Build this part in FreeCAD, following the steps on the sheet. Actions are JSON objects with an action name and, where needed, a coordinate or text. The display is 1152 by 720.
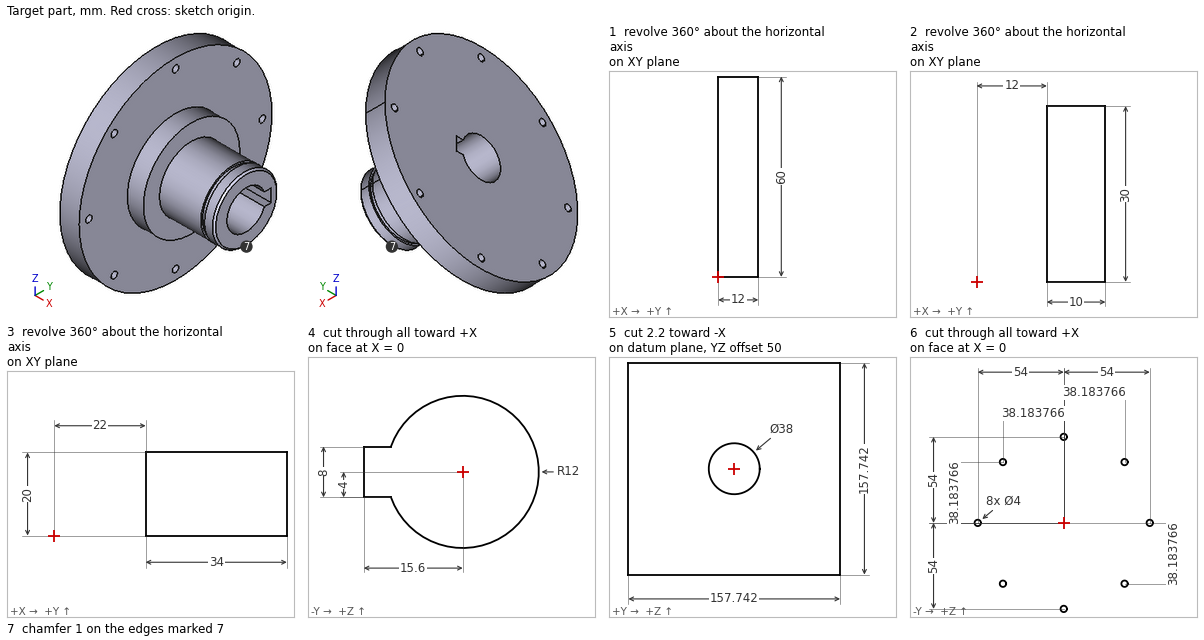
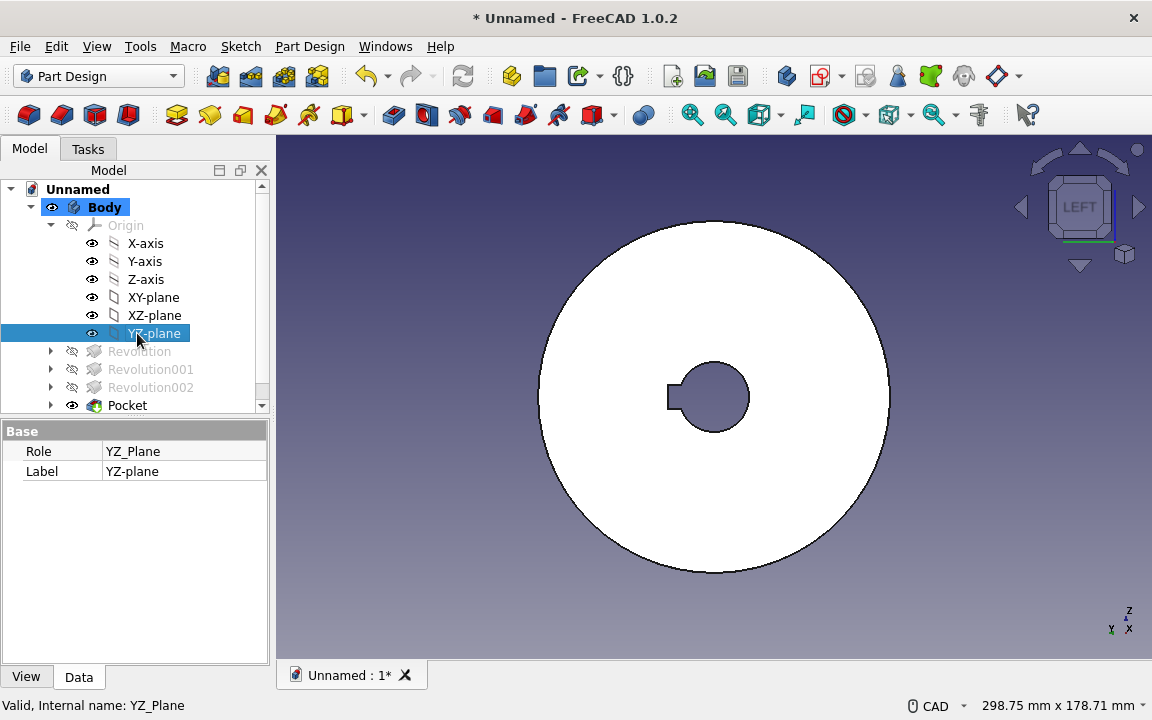
{"action": "left_click", "coordinate": [996, 76]}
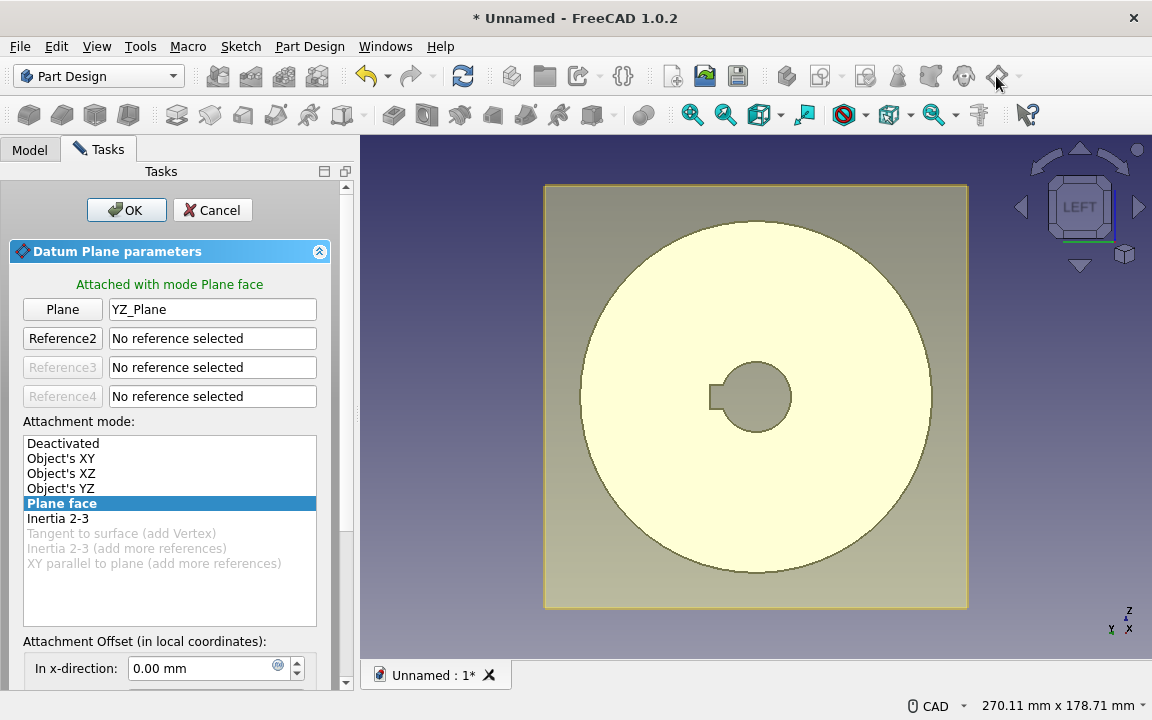
{"action": "scroll", "coordinate": [346, 436], "scroll_direction": "down", "scroll_amount": 2}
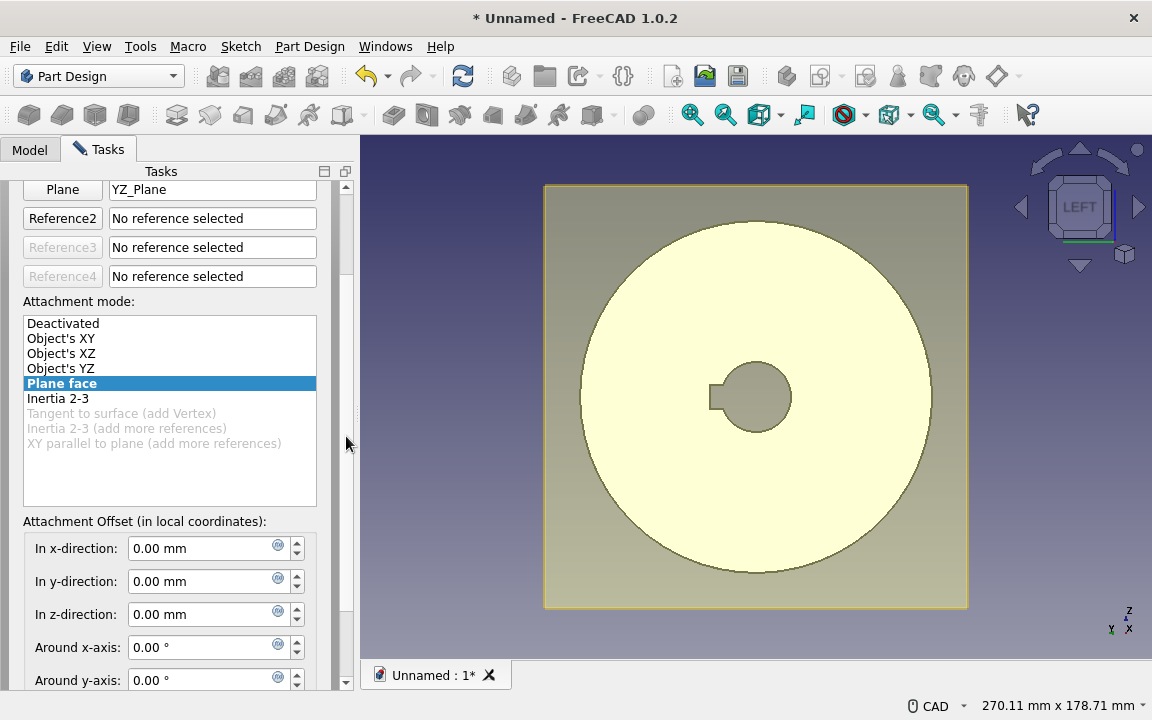
{"action": "triple_click", "coordinate": [210, 614]}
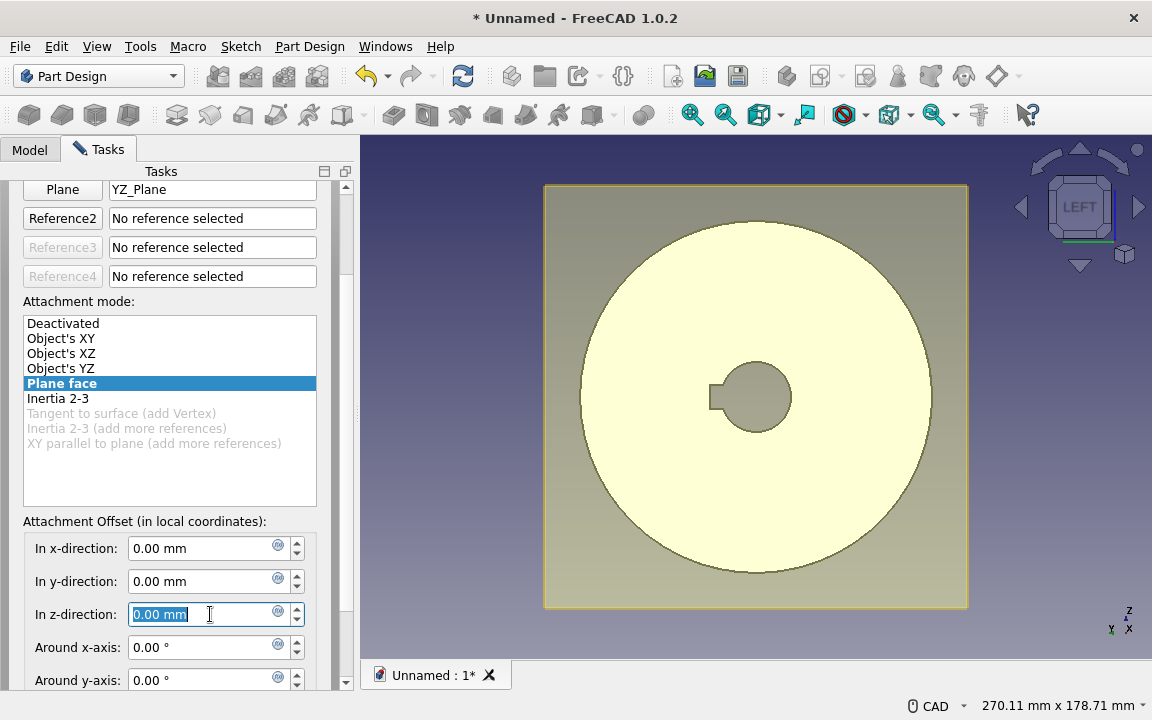
{"action": "type", "text": "50"}
{"action": "key", "text": "Tab"}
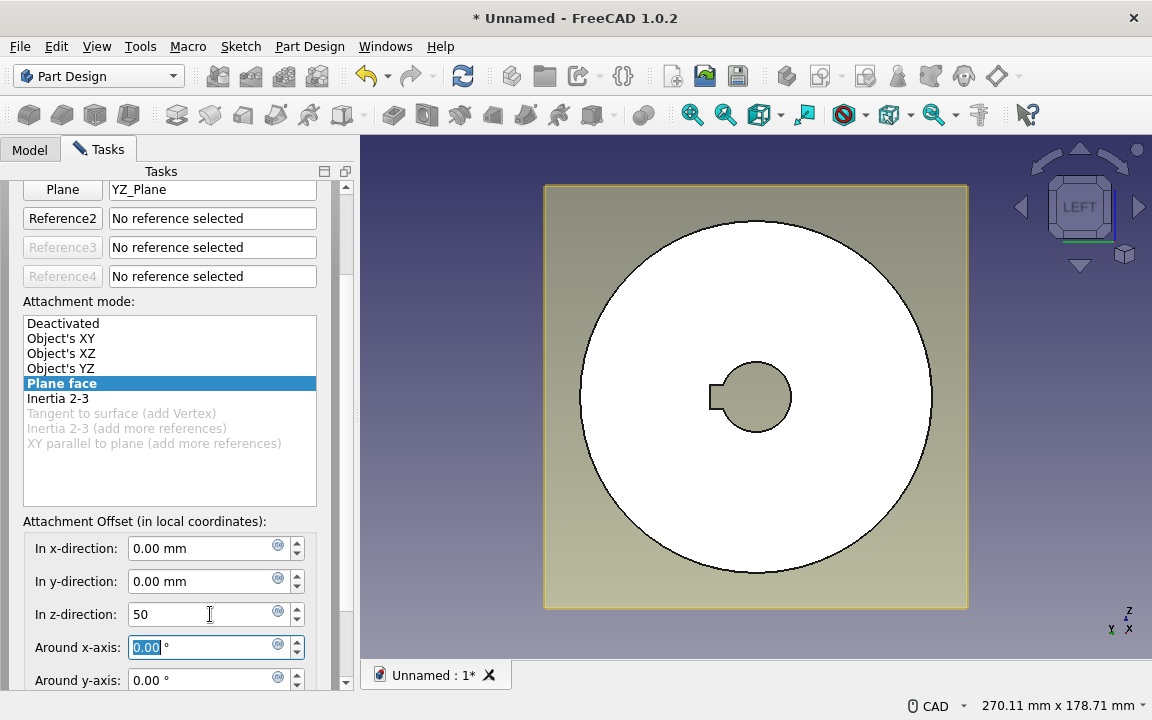
{"action": "scroll", "coordinate": [346, 436], "scroll_direction": "up", "scroll_amount": 3}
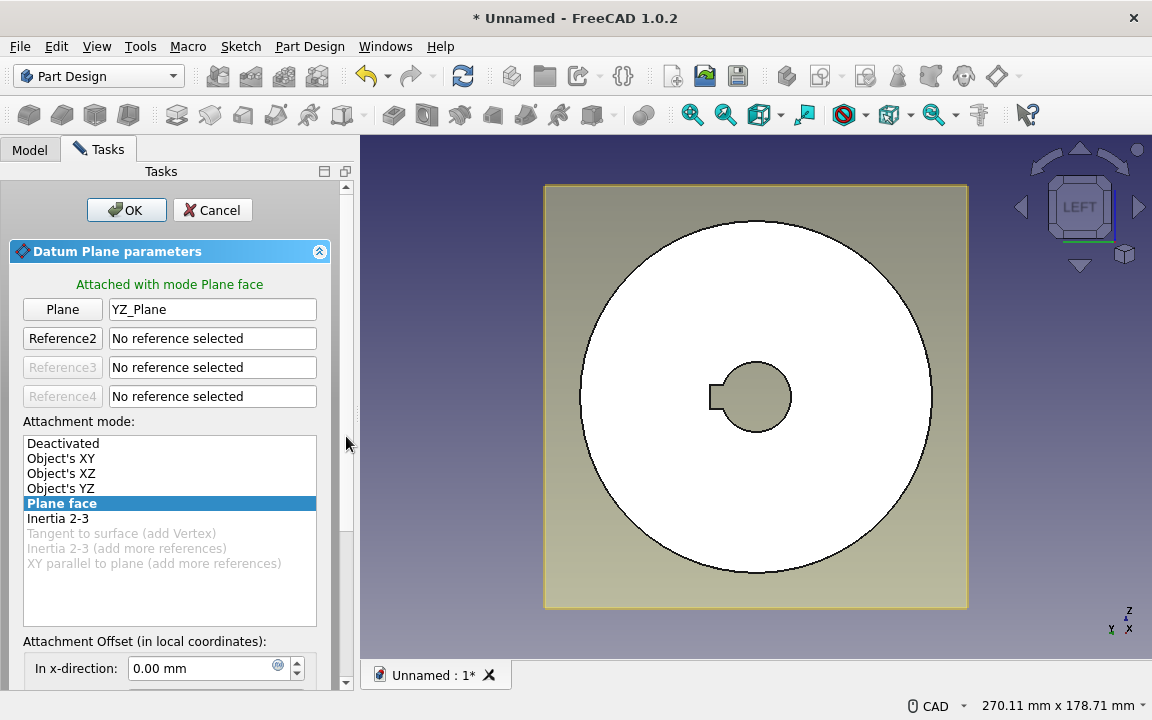
{"action": "left_click", "coordinate": [127, 210]}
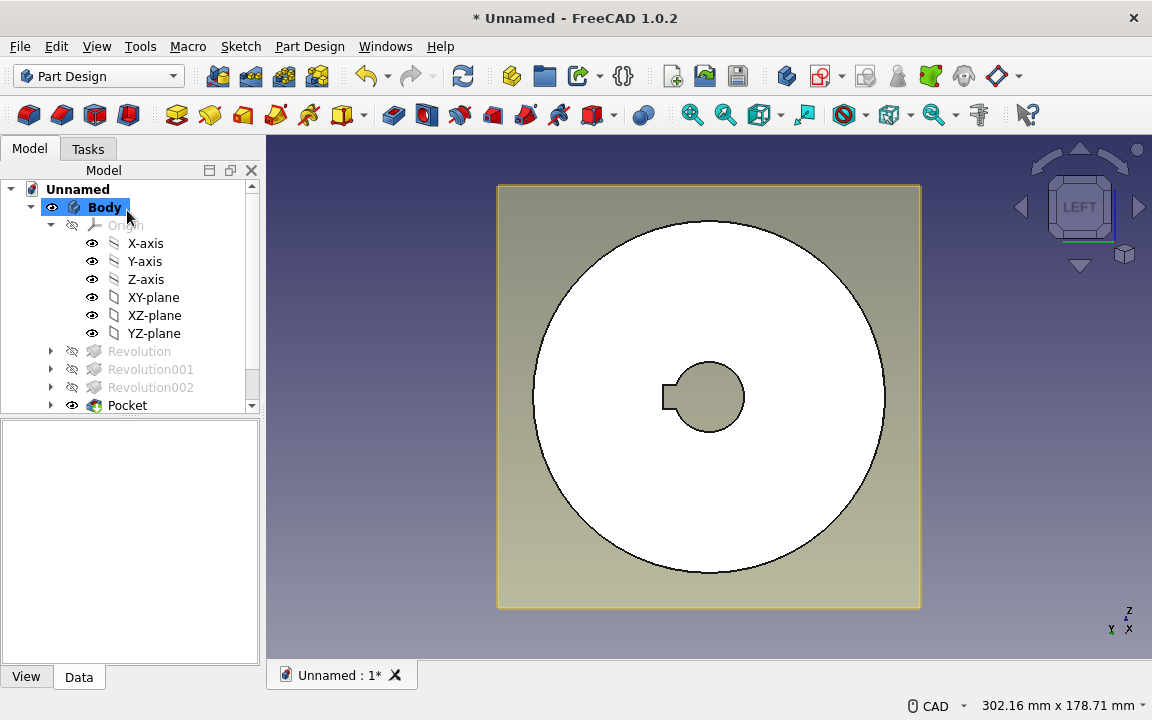
{"action": "scroll", "coordinate": [101, 293], "scroll_direction": "down", "scroll_amount": 3}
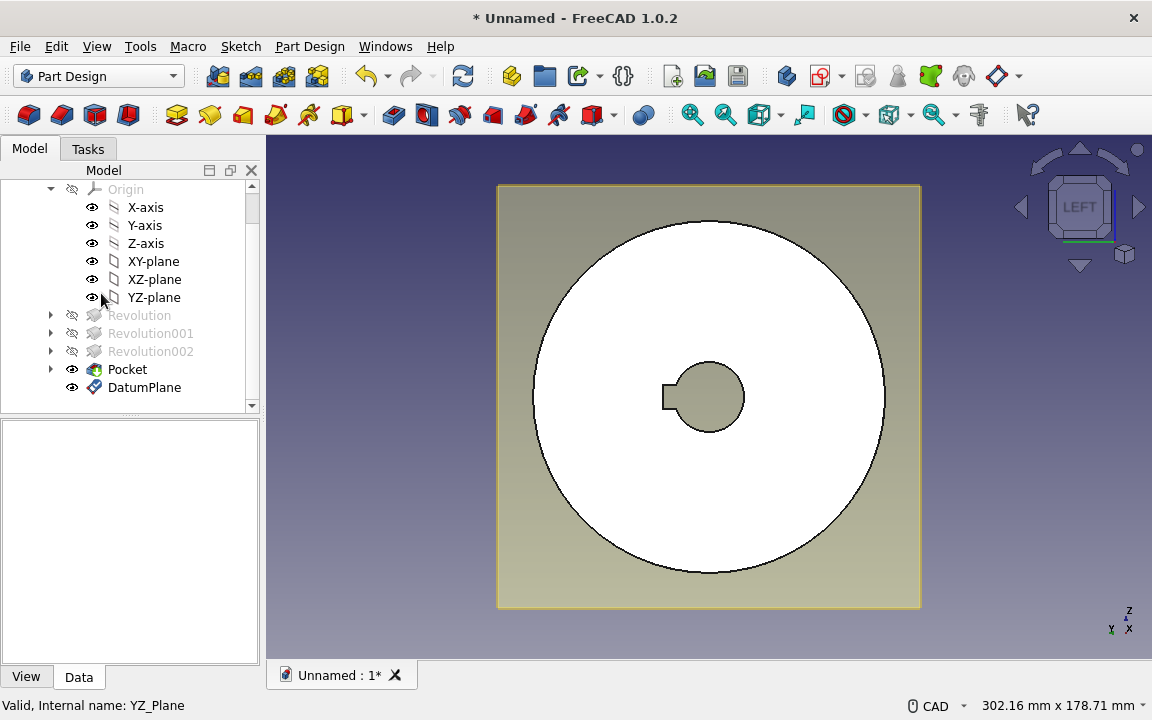
{"action": "left_click", "coordinate": [117, 387]}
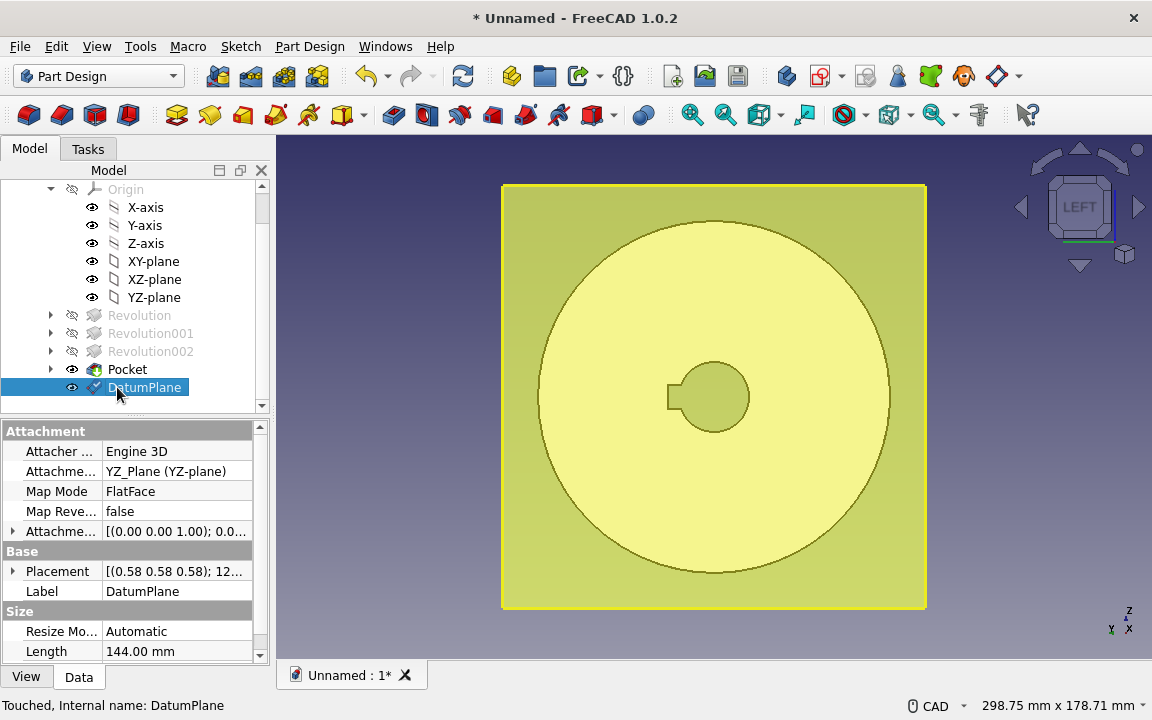
{"action": "left_click", "coordinate": [820, 76]}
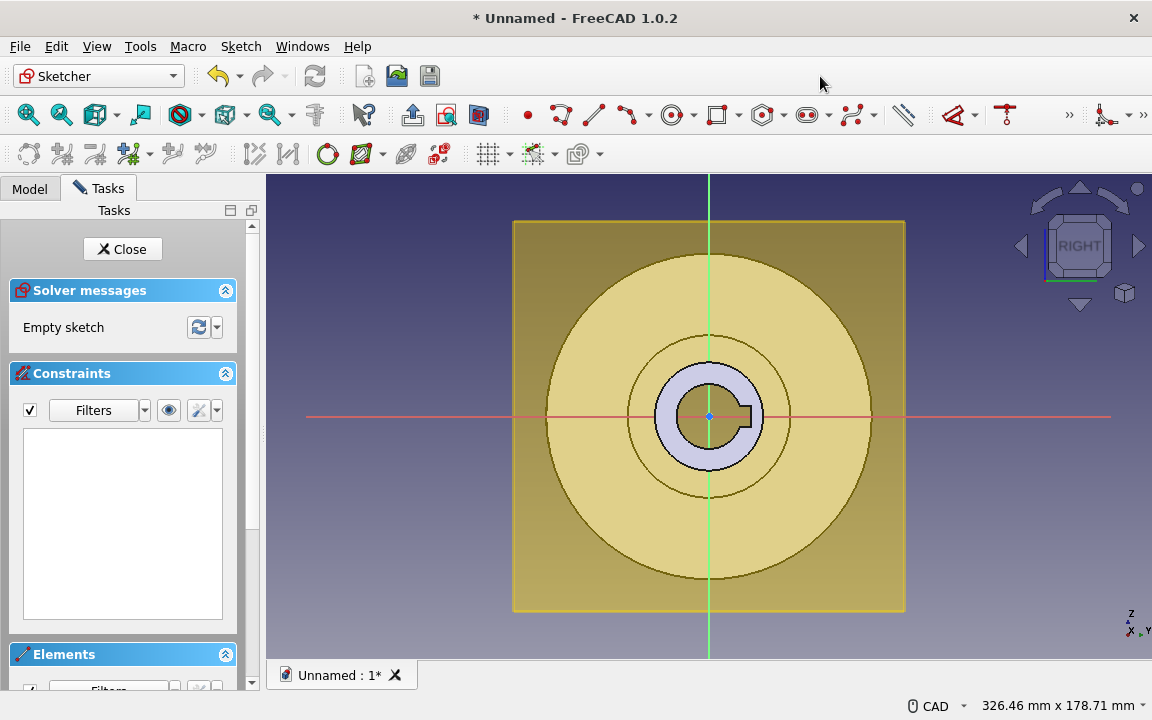
{"action": "left_click", "coordinate": [479, 116]}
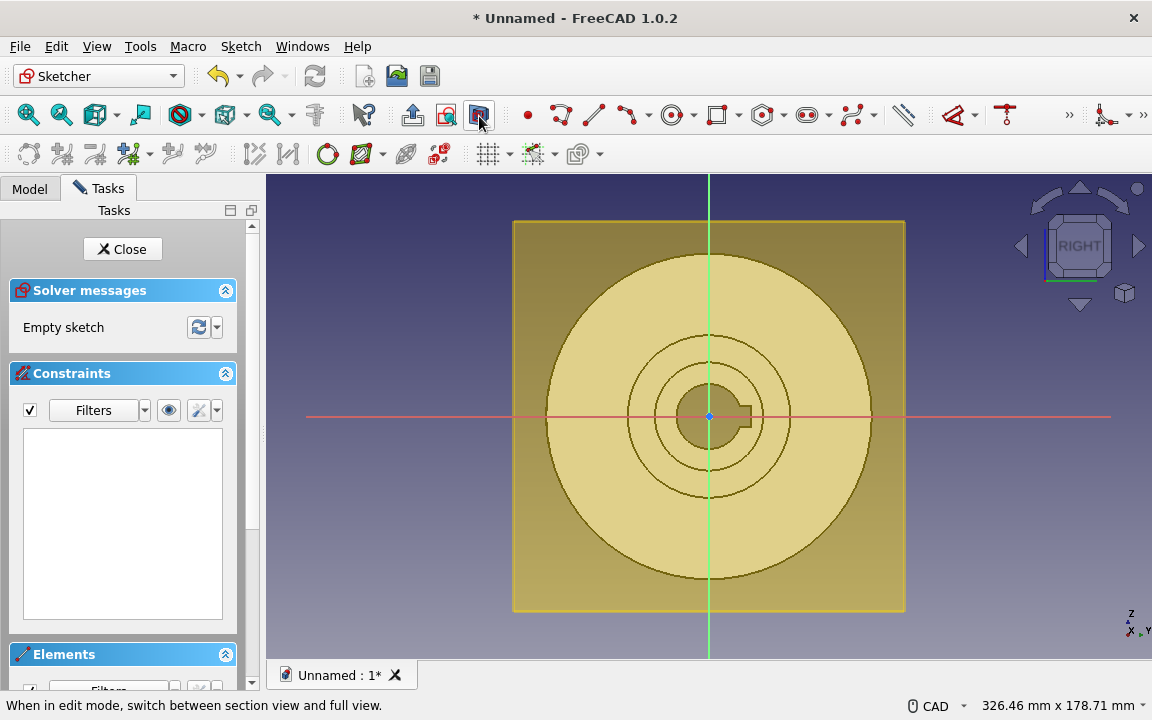
{"action": "scroll", "coordinate": [501, 416], "scroll_direction": "down", "scroll_amount": 2}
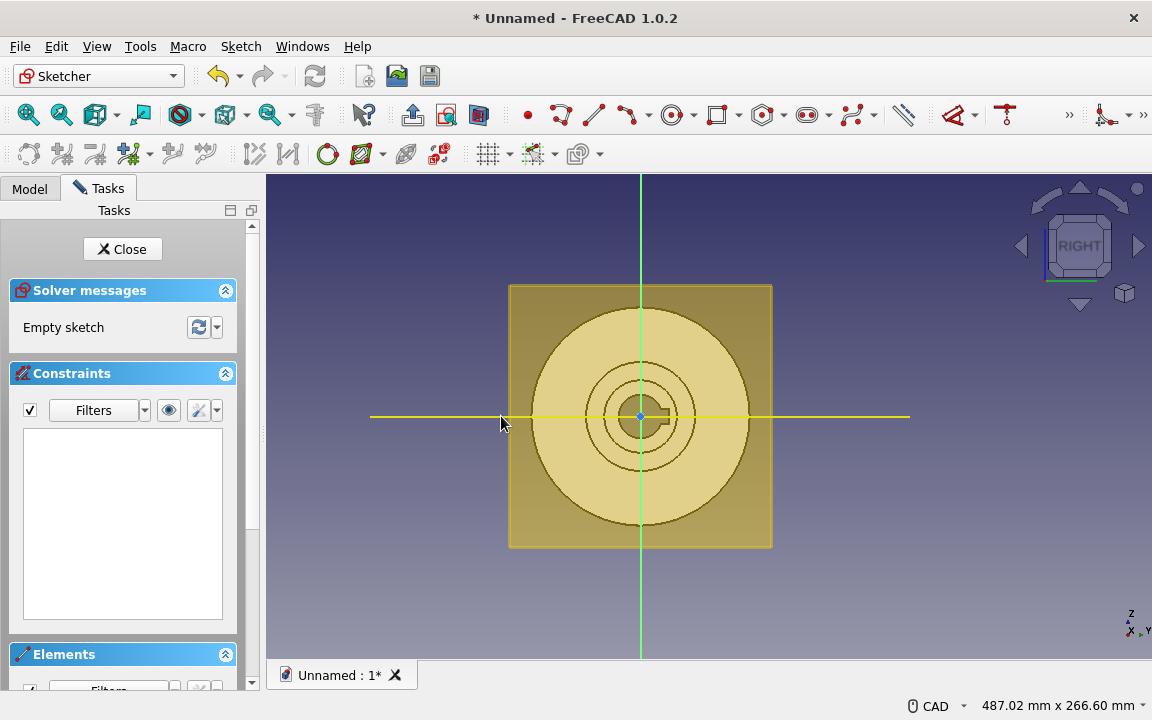
{"action": "key", "text": "g v"}